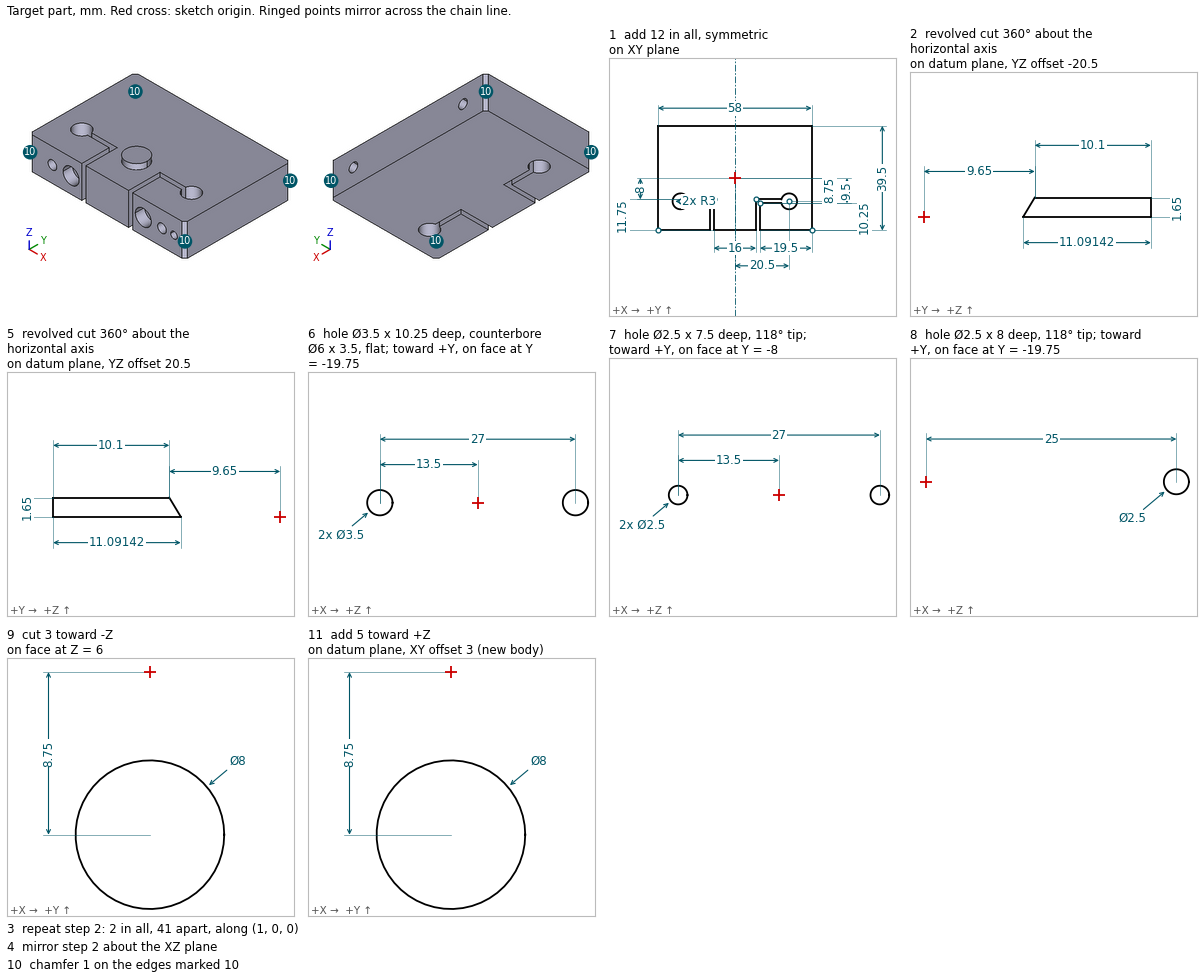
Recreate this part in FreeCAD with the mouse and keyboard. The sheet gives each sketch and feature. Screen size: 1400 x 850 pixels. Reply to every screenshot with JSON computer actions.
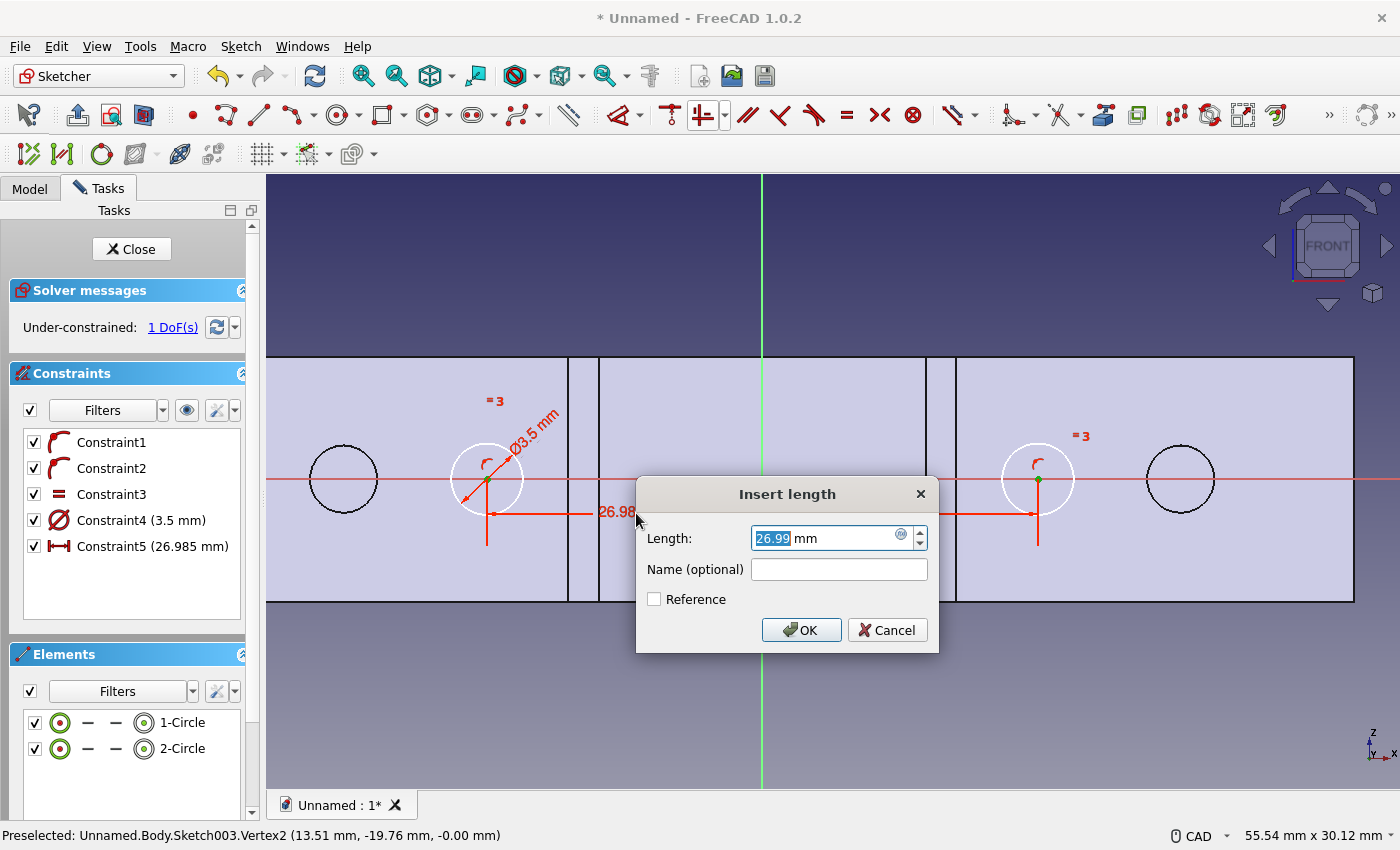
{"action": "type", "text": "27"}
{"action": "key", "text": "Return"}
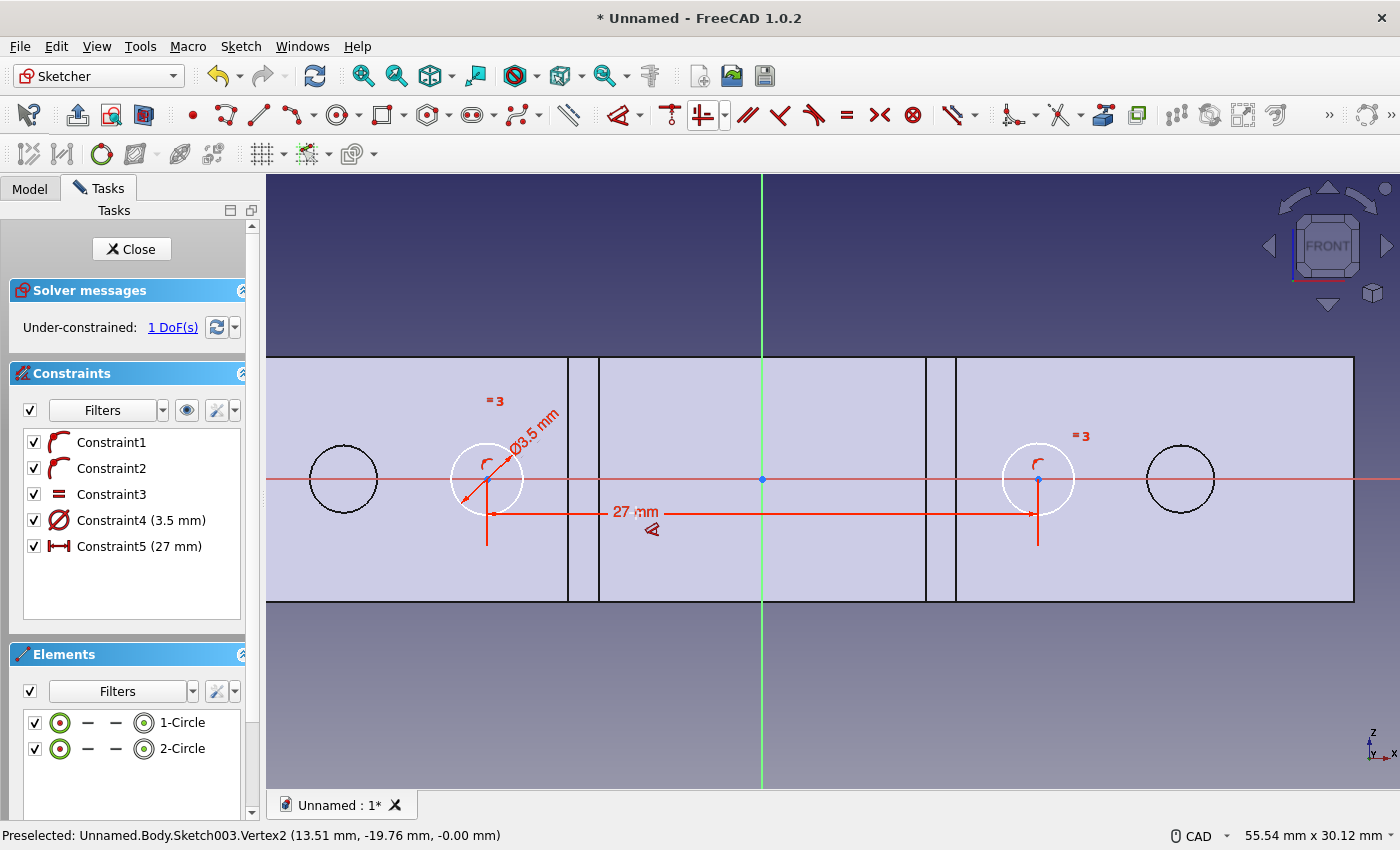
{"action": "left_click", "coordinate": [487, 479]}
{"action": "left_click", "coordinate": [561, 513]}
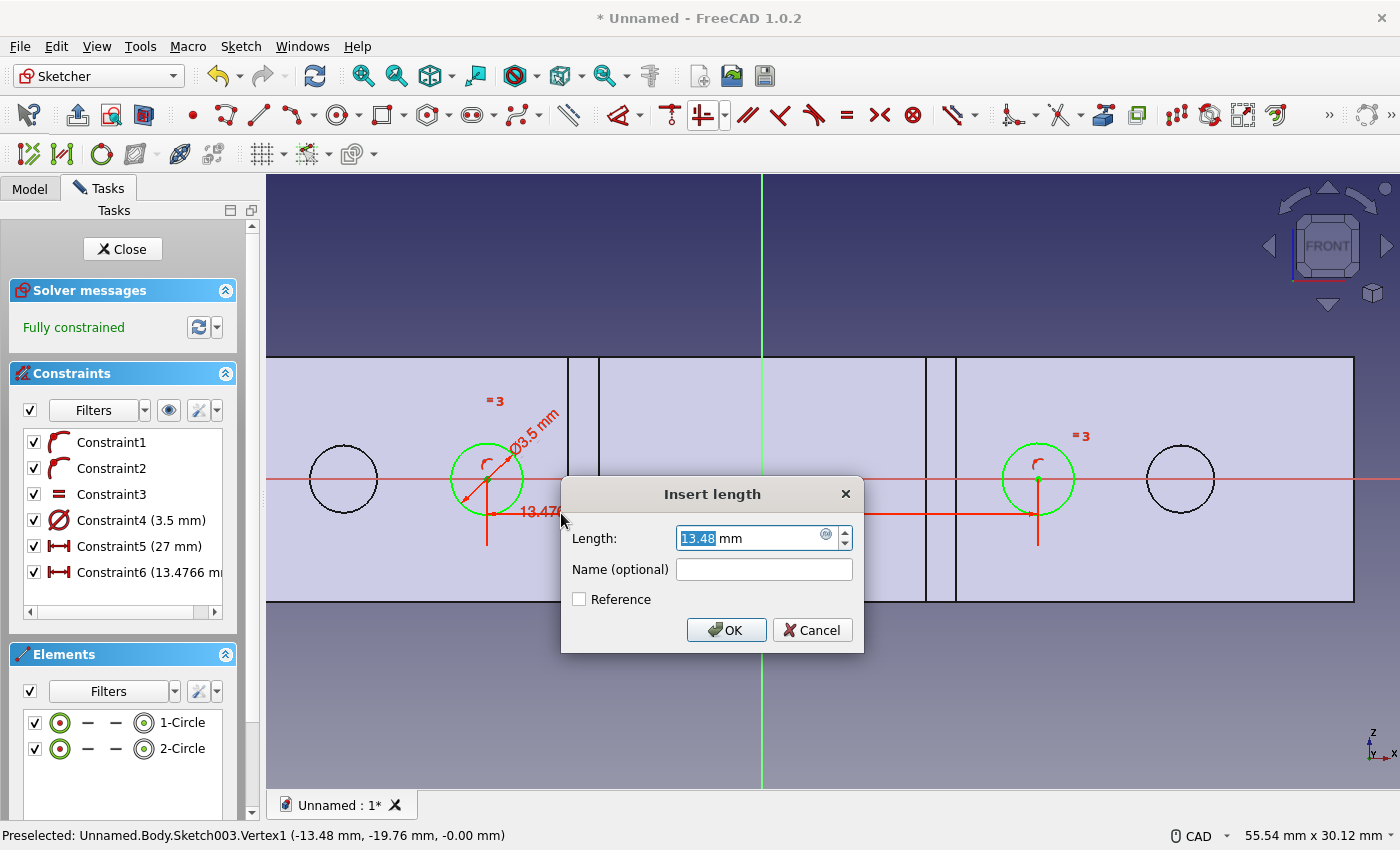
{"action": "type", "text": "13.5"}
{"action": "key", "text": "Return"}
{"action": "key", "text": "Escape"}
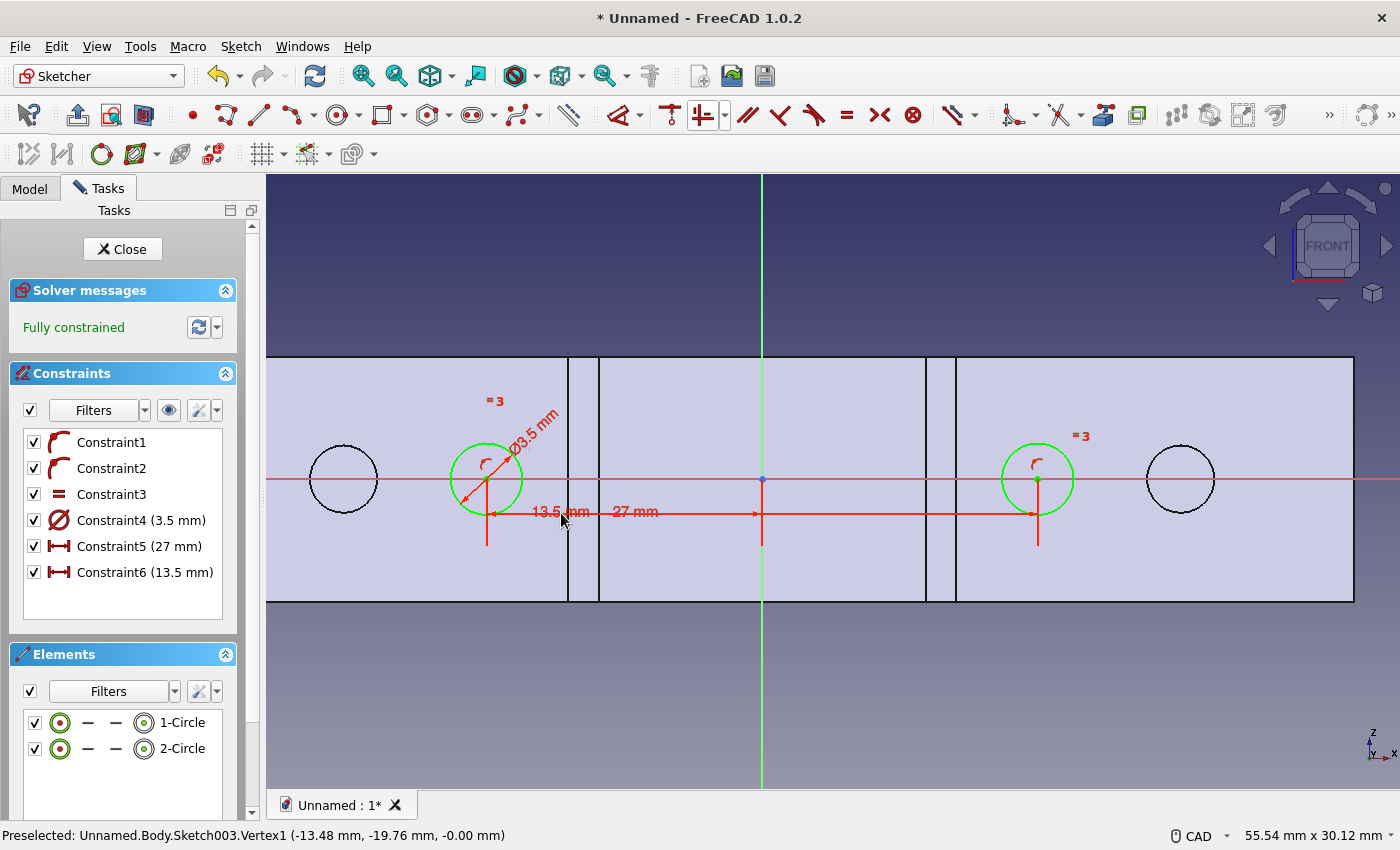
{"action": "left_click", "coordinate": [123, 249]}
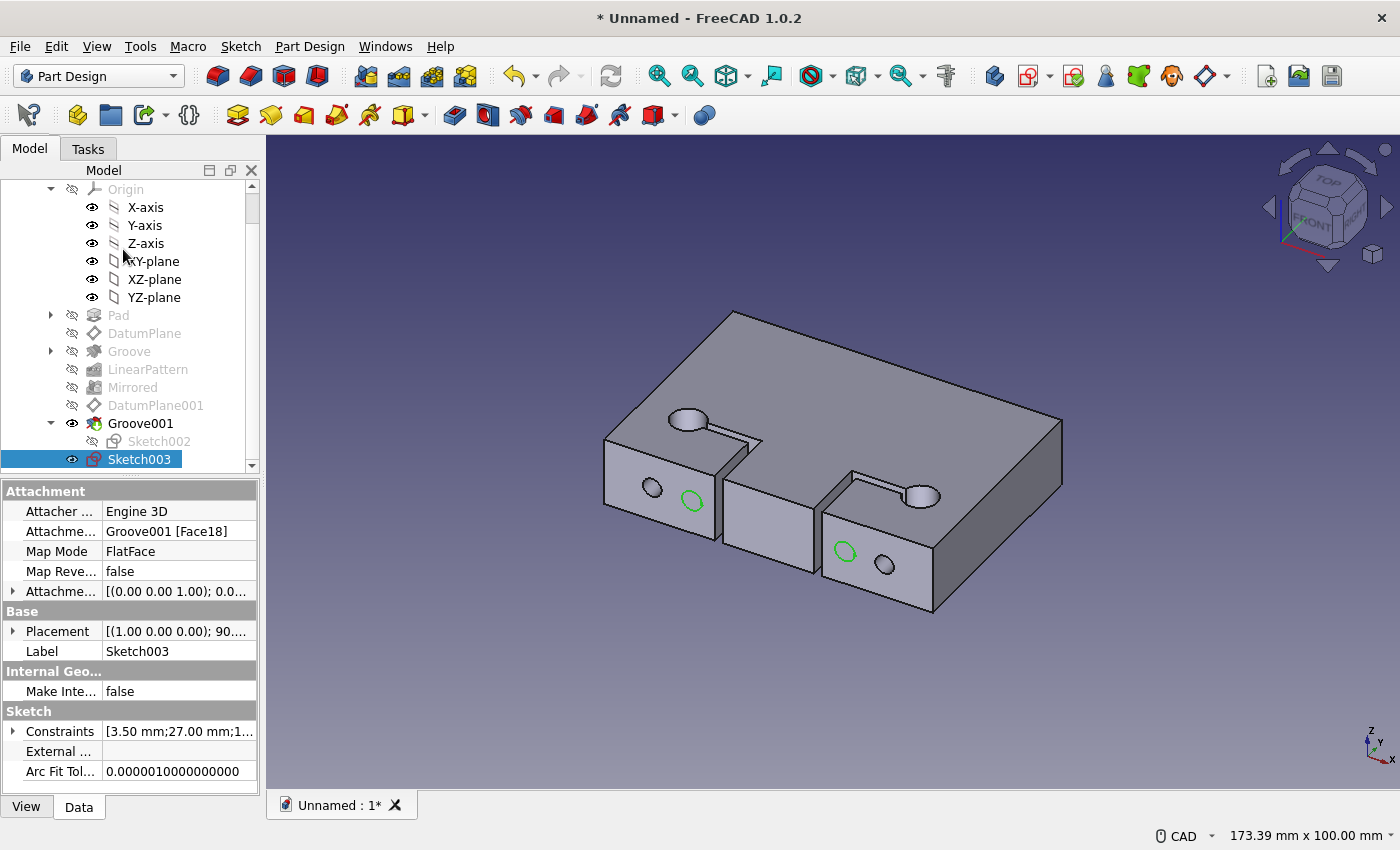
{"action": "left_click", "coordinate": [488, 116]}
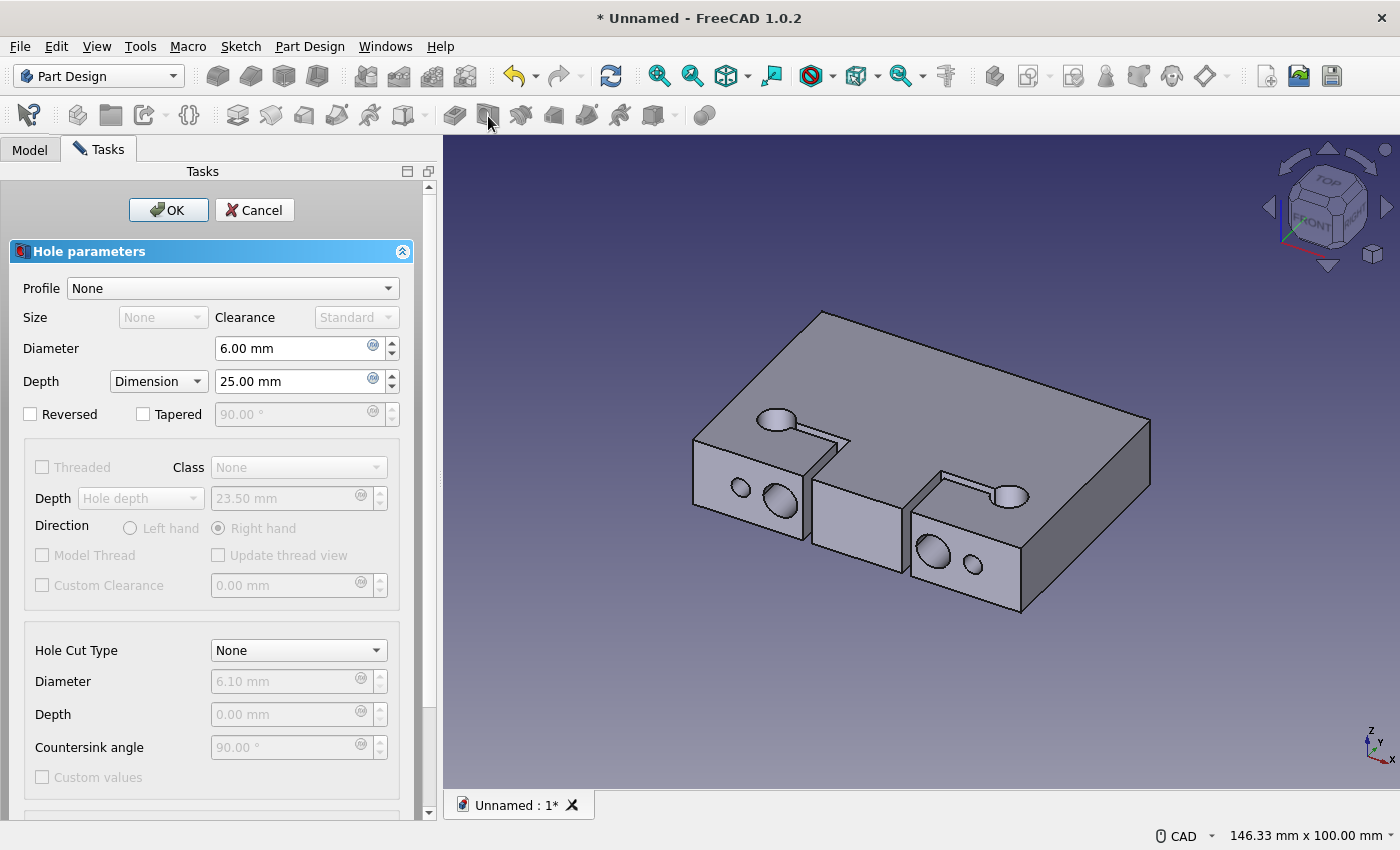
{"action": "triple_click", "coordinate": [300, 348]}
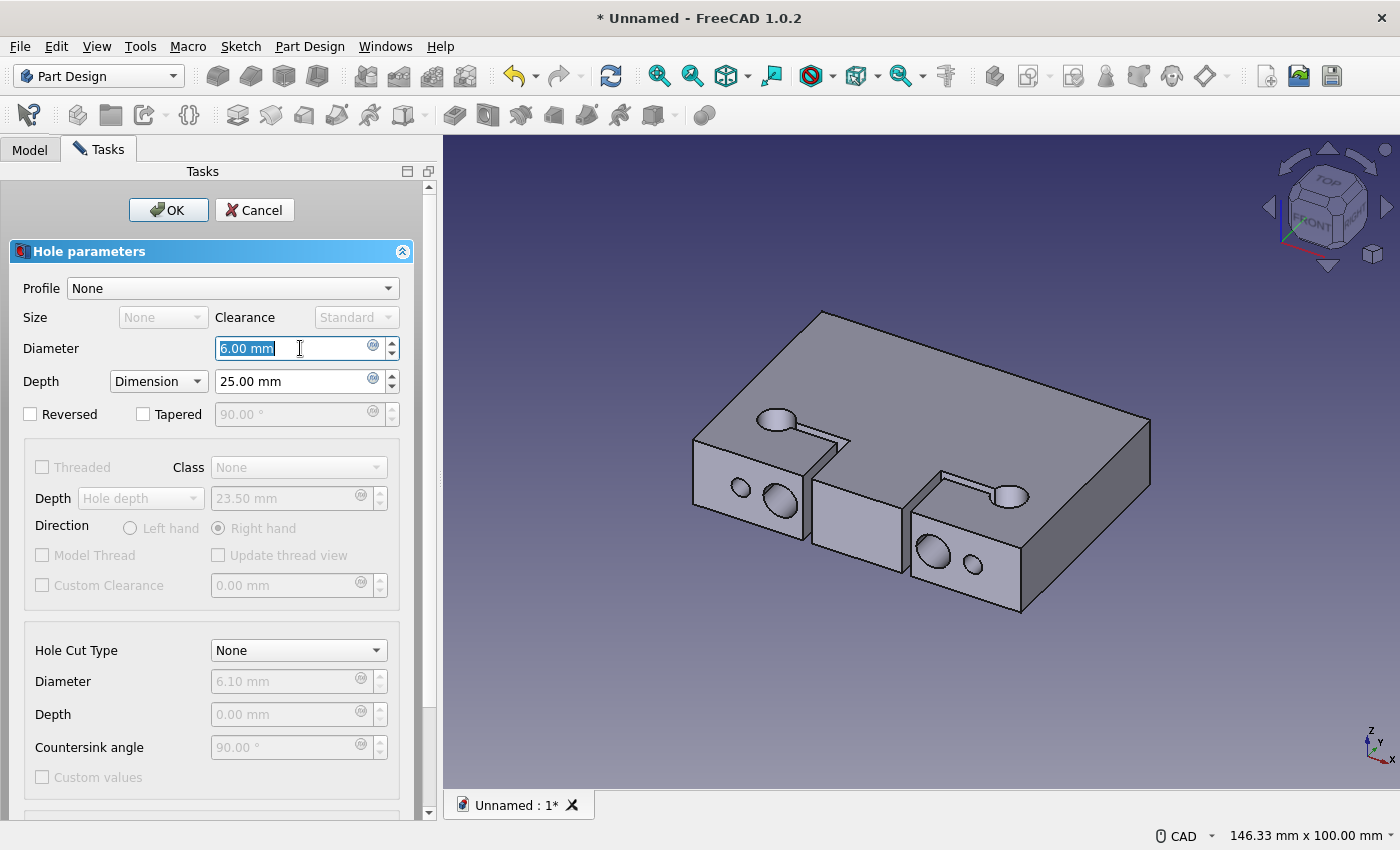
{"action": "type", "text": "3.5"}
{"action": "key", "text": "Tab"}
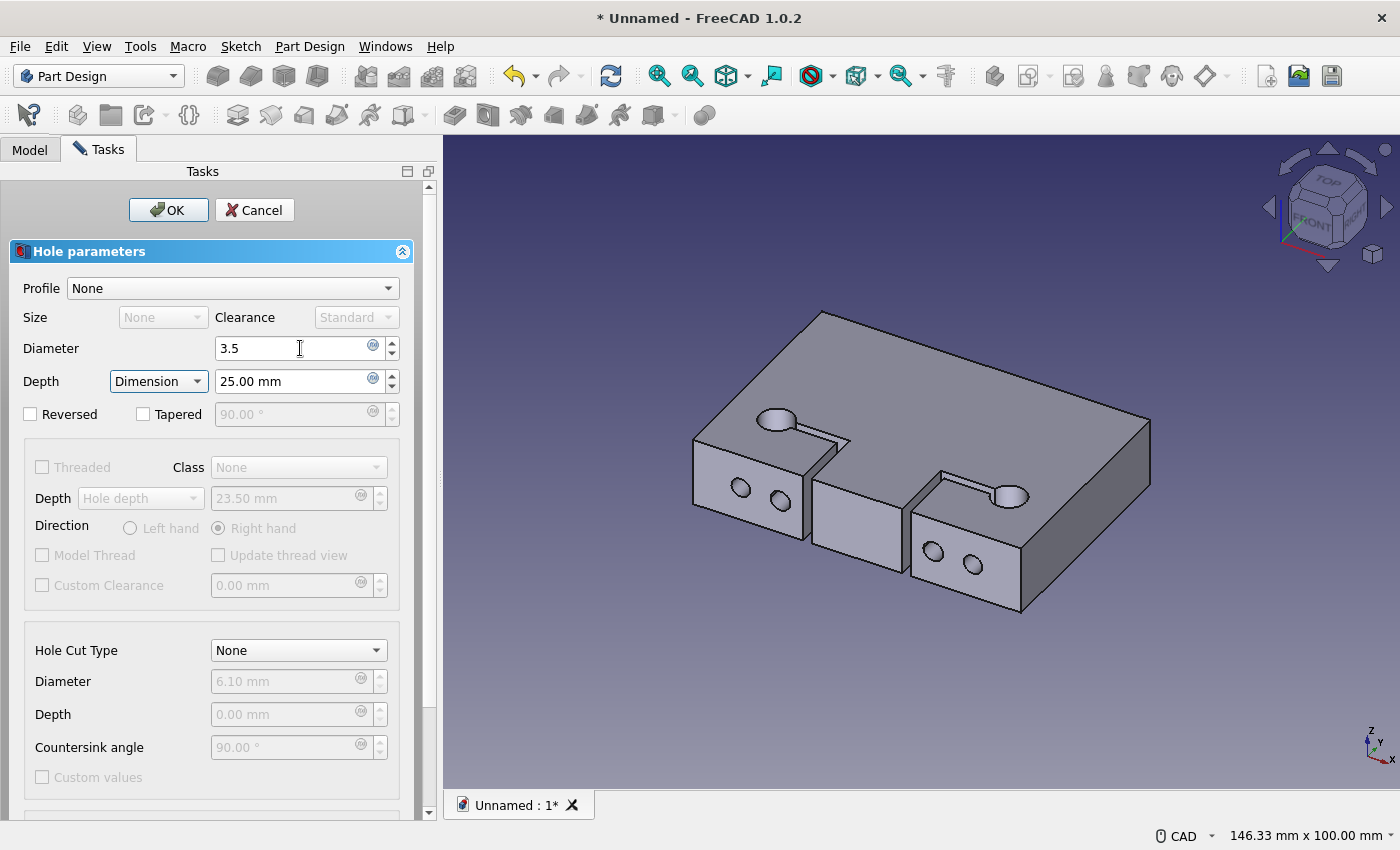
{"action": "triple_click", "coordinate": [300, 382]}